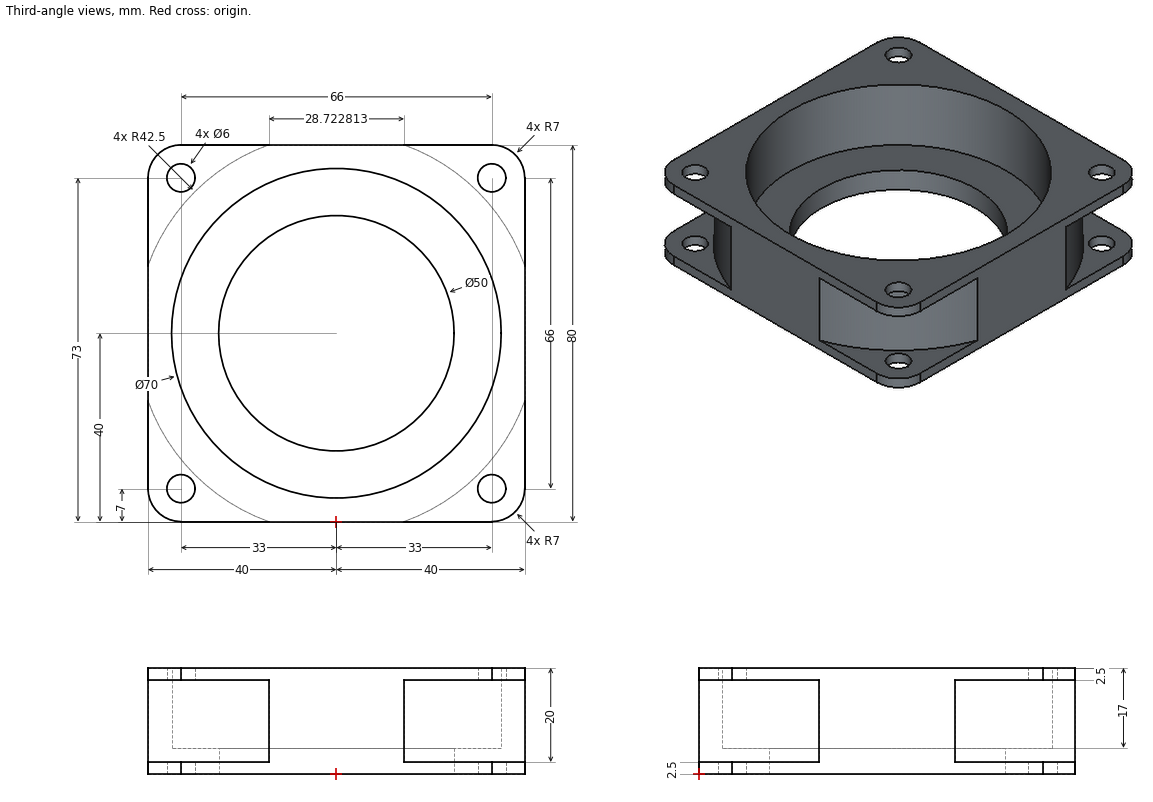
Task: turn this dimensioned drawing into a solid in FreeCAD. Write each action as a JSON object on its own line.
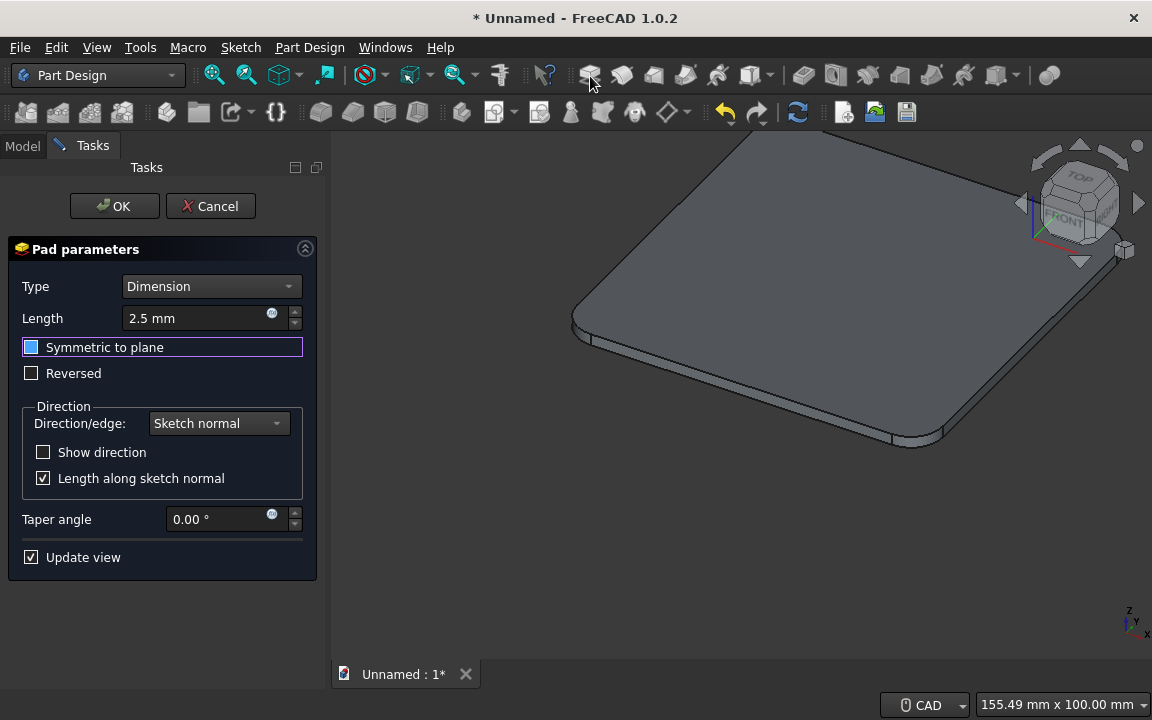
{"action": "left_click", "coordinate": [115, 206]}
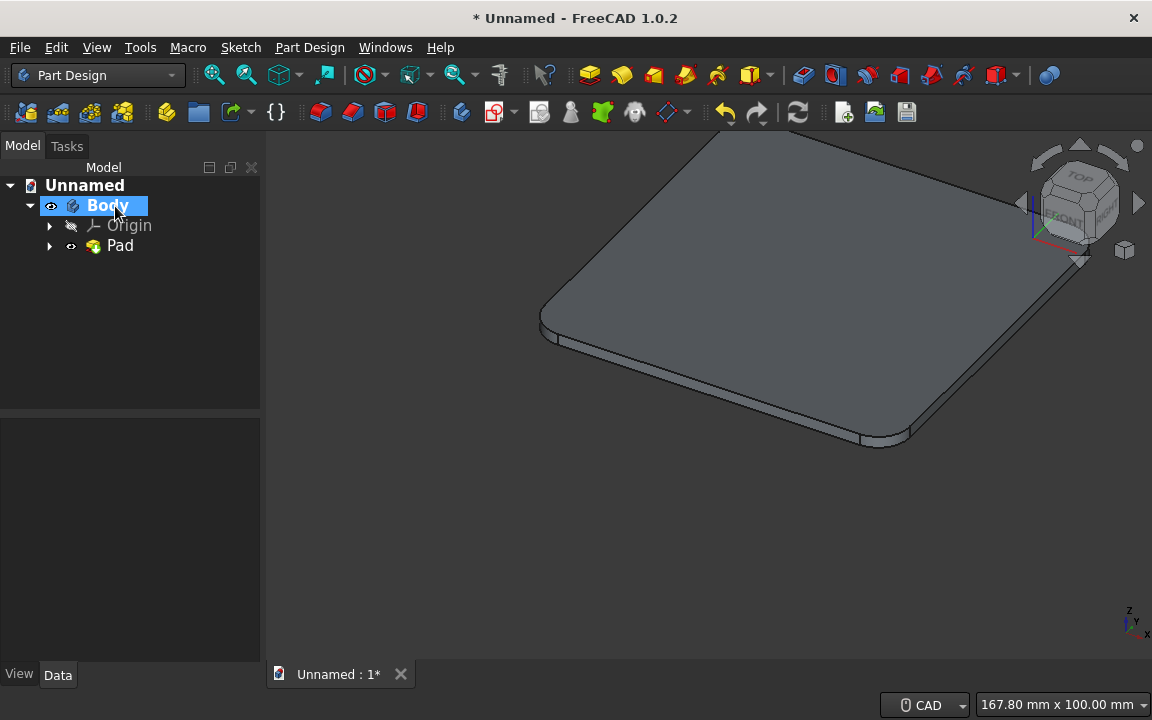
{"action": "key", "text": "v f"}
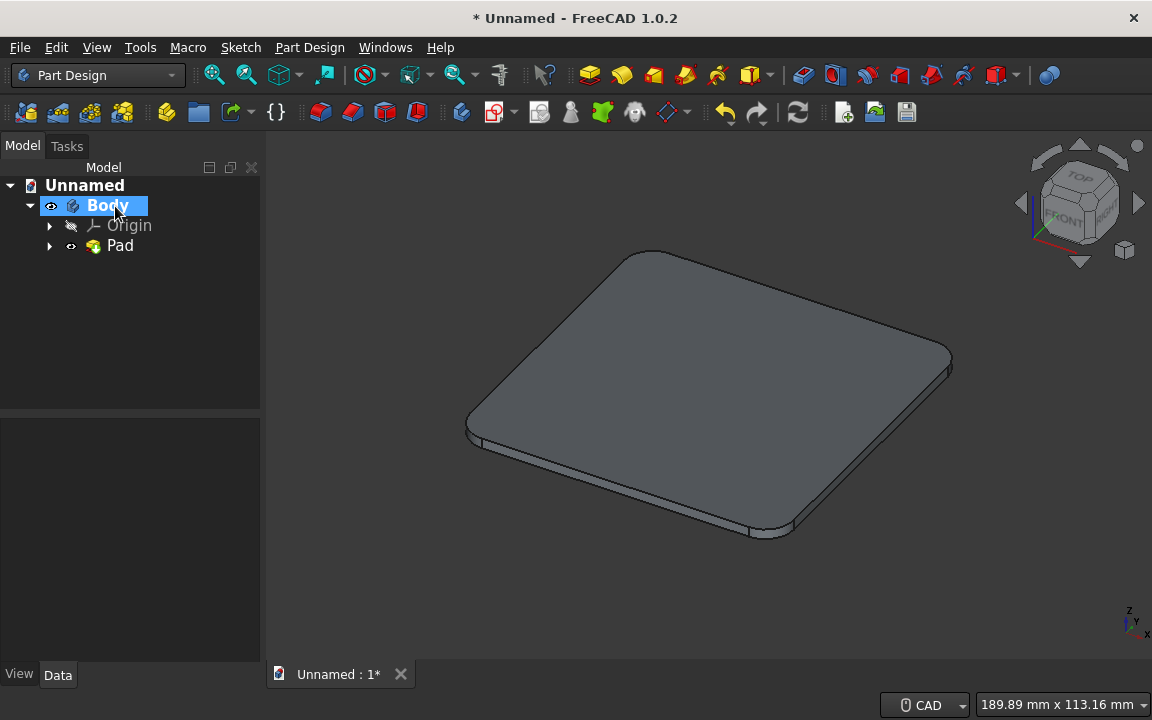
{"action": "left_click", "coordinate": [709, 389]}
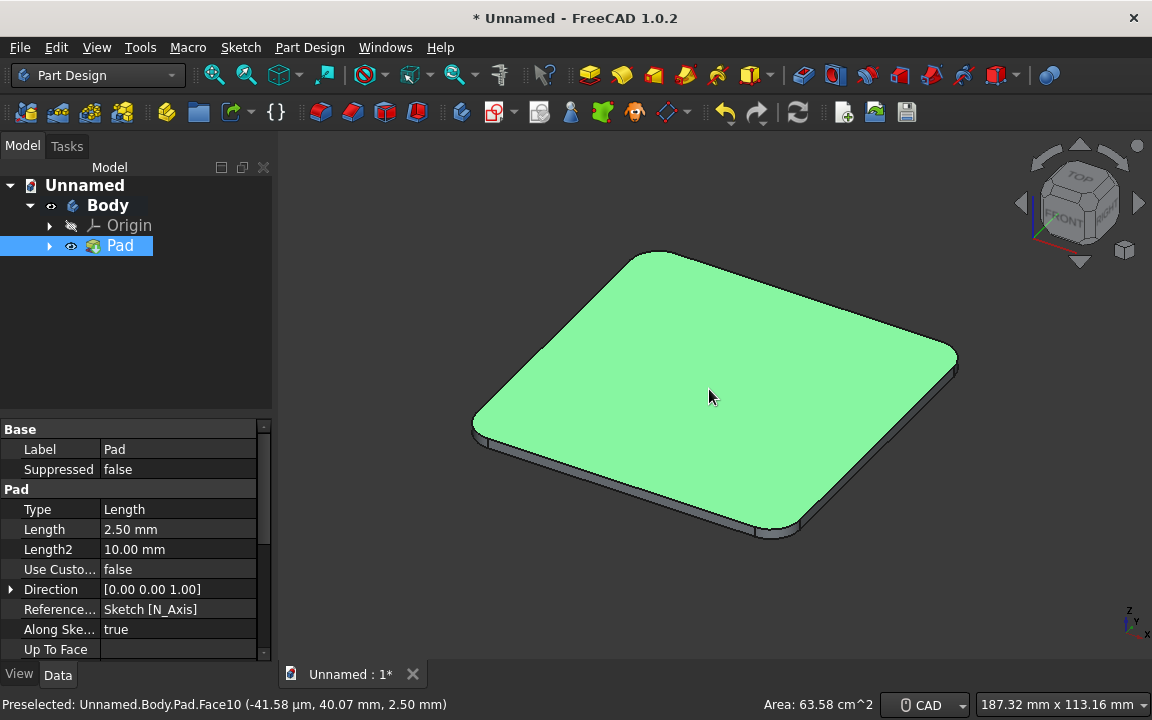
{"action": "left_click", "coordinate": [494, 112]}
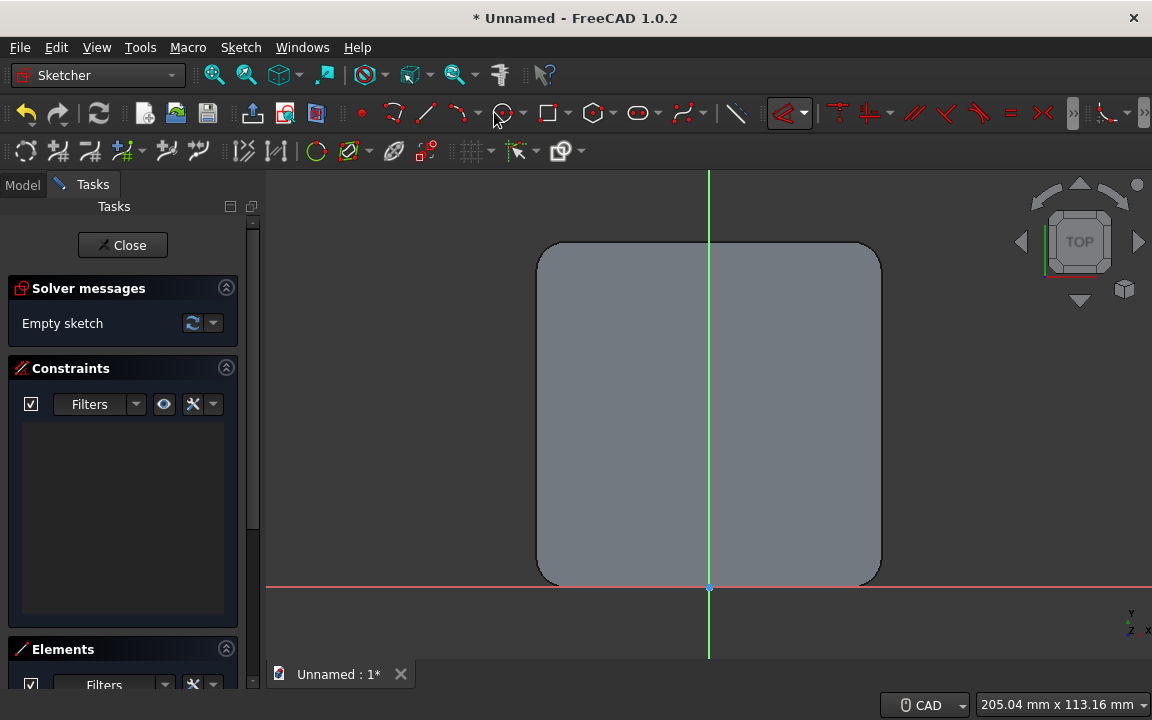
{"action": "key", "text": "g c"}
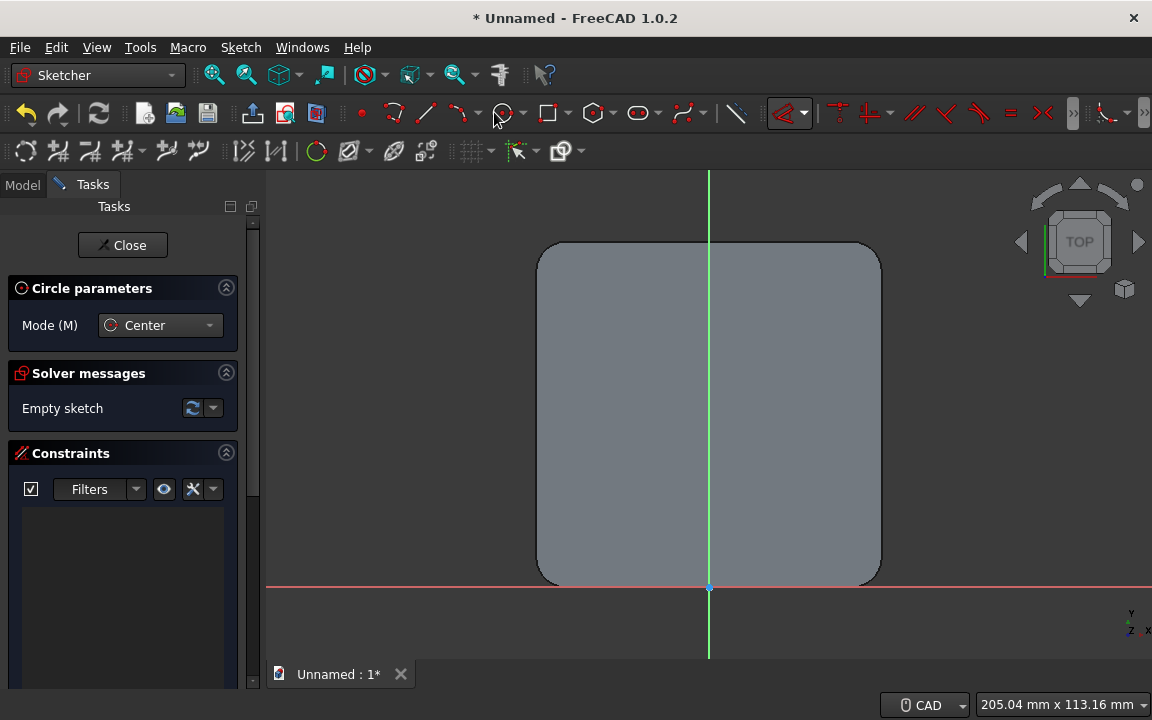
{"action": "left_click", "coordinate": [709, 414]}
{"action": "mouse_move", "coordinate": [816, 308]}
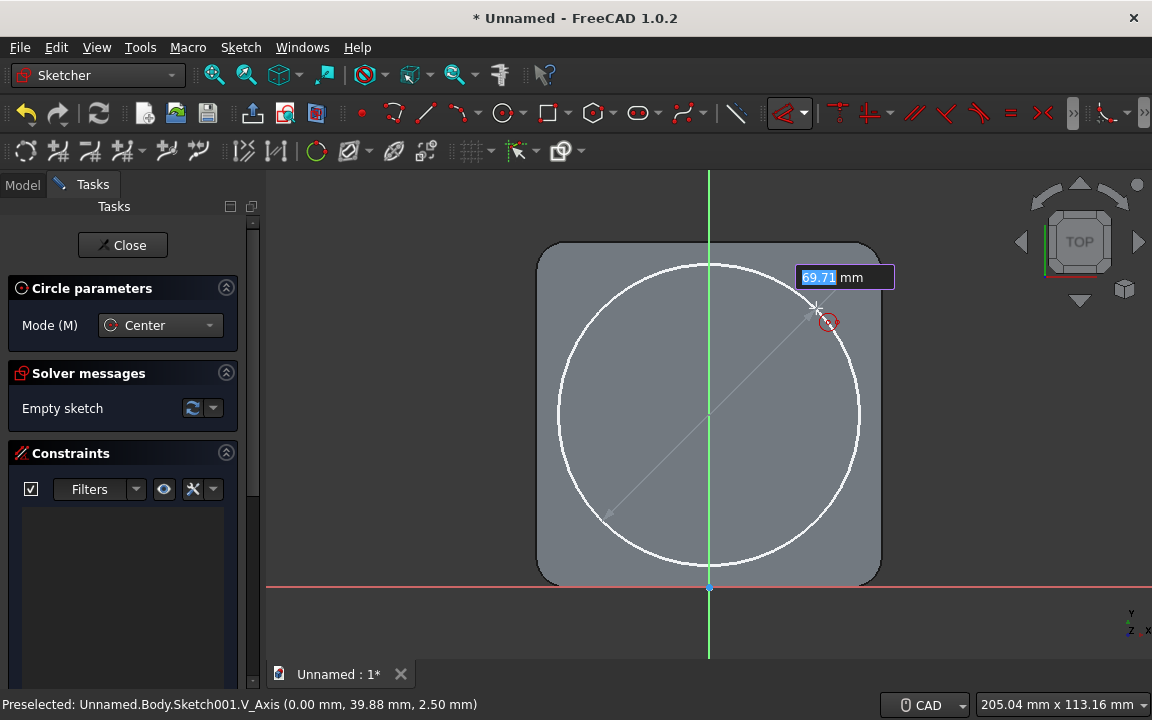
{"action": "type", "text": "70"}
{"action": "key", "text": "Return"}
{"action": "key", "text": "Escape"}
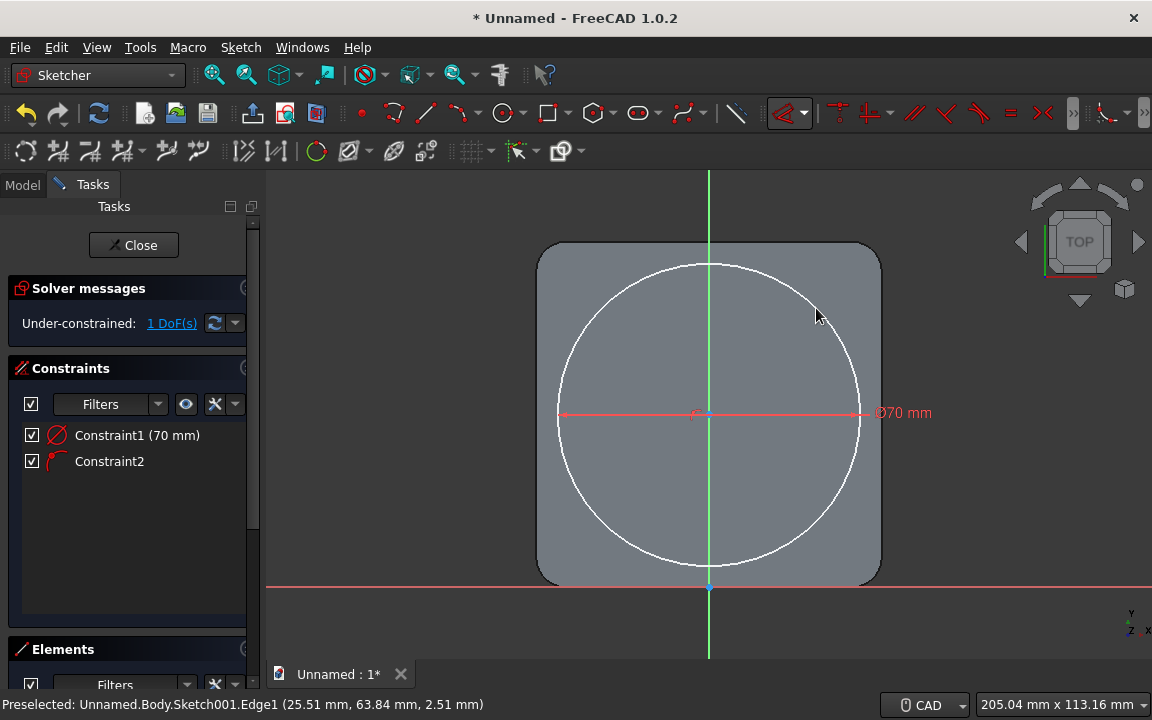
{"action": "key", "text": "d"}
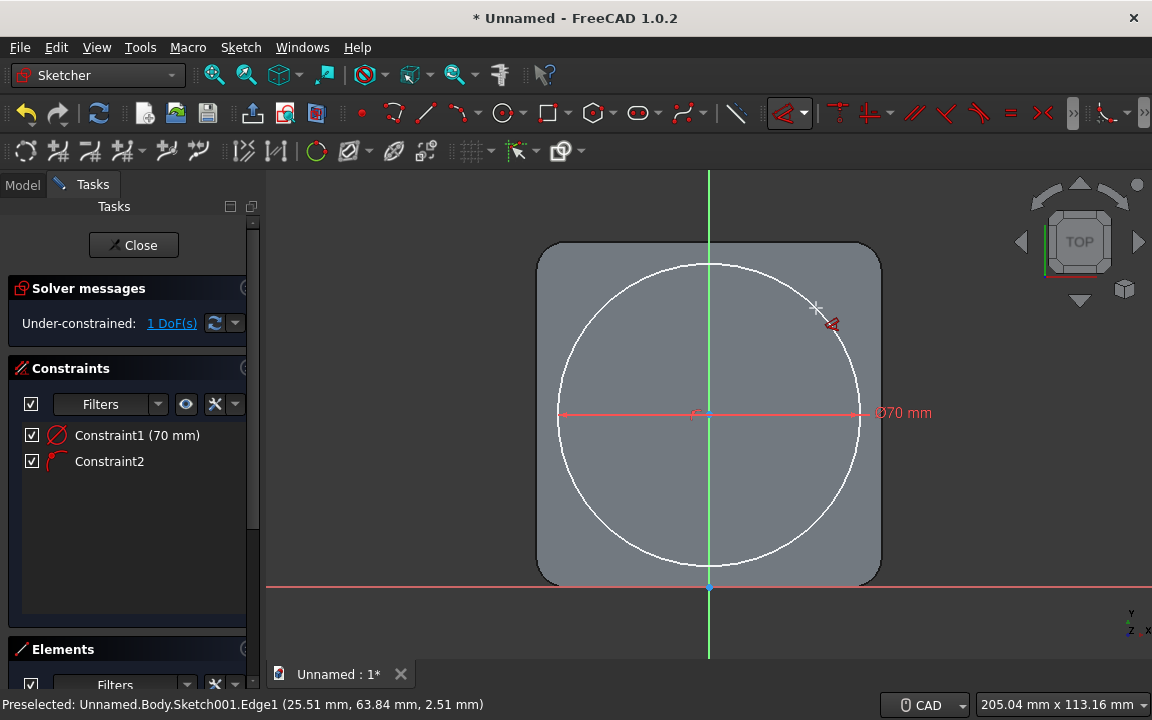
{"action": "left_click", "coordinate": [709, 415]}
{"action": "left_click", "coordinate": [743, 501]}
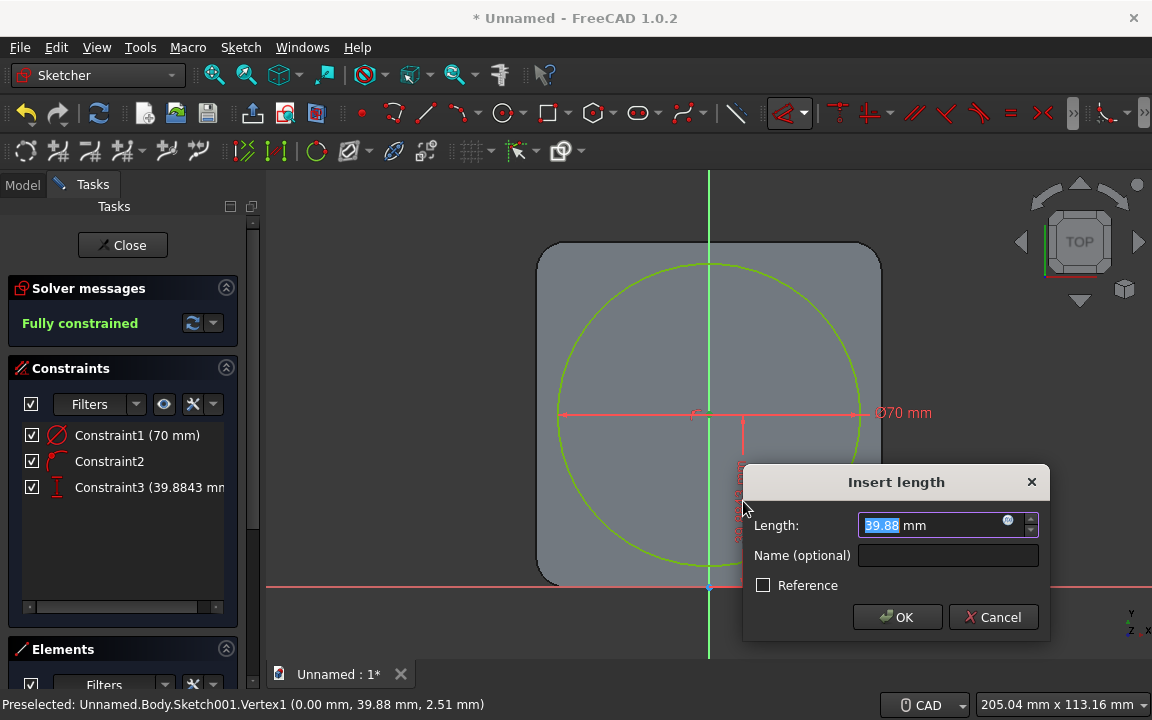
{"action": "type", "text": "40"}
{"action": "key", "text": "Return"}
{"action": "key", "text": "Escape"}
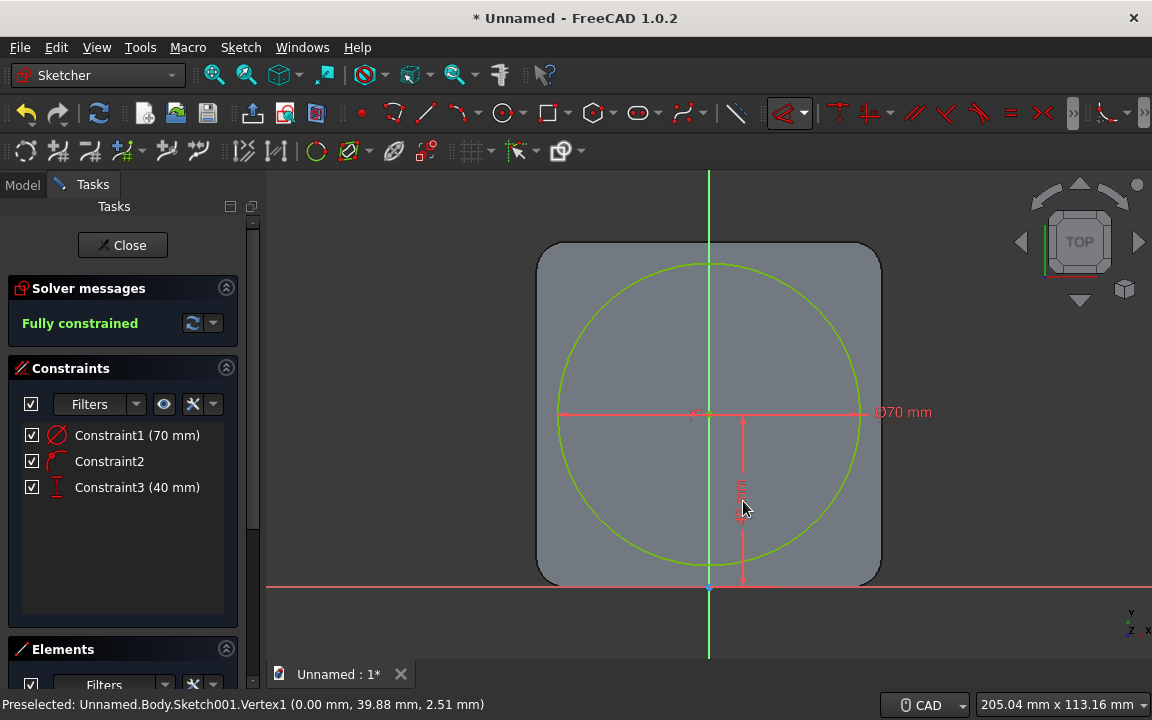
{"action": "left_click", "coordinate": [123, 245]}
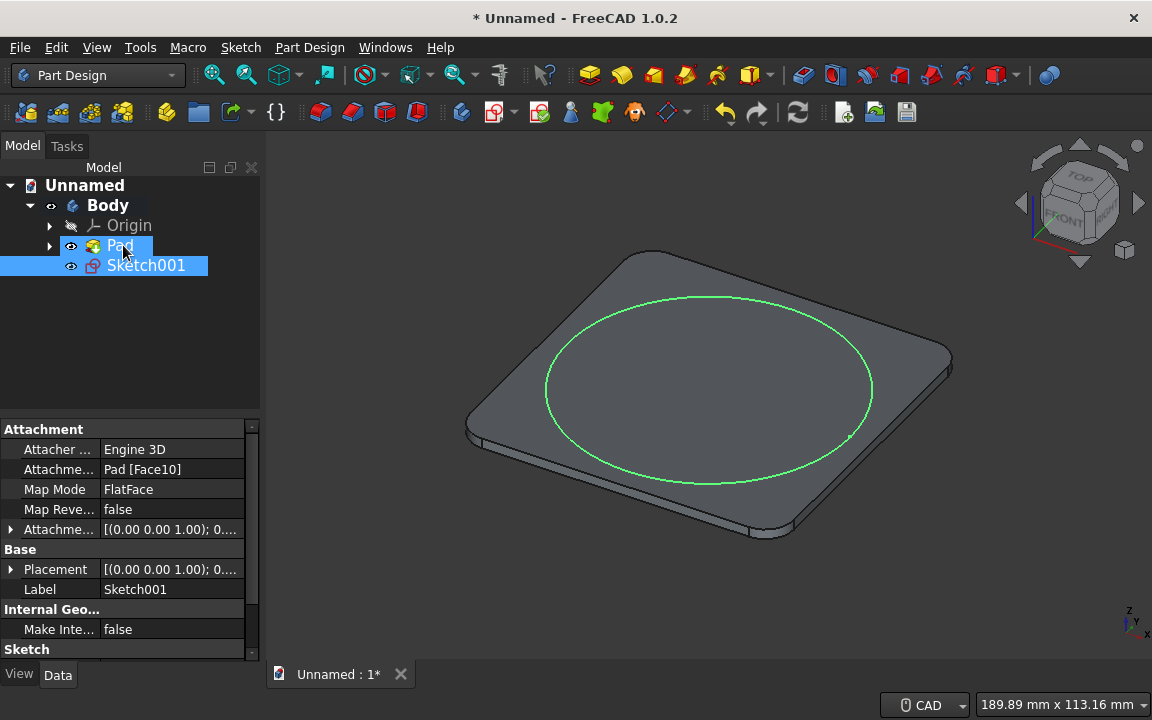
{"action": "left_click", "coordinate": [590, 76]}